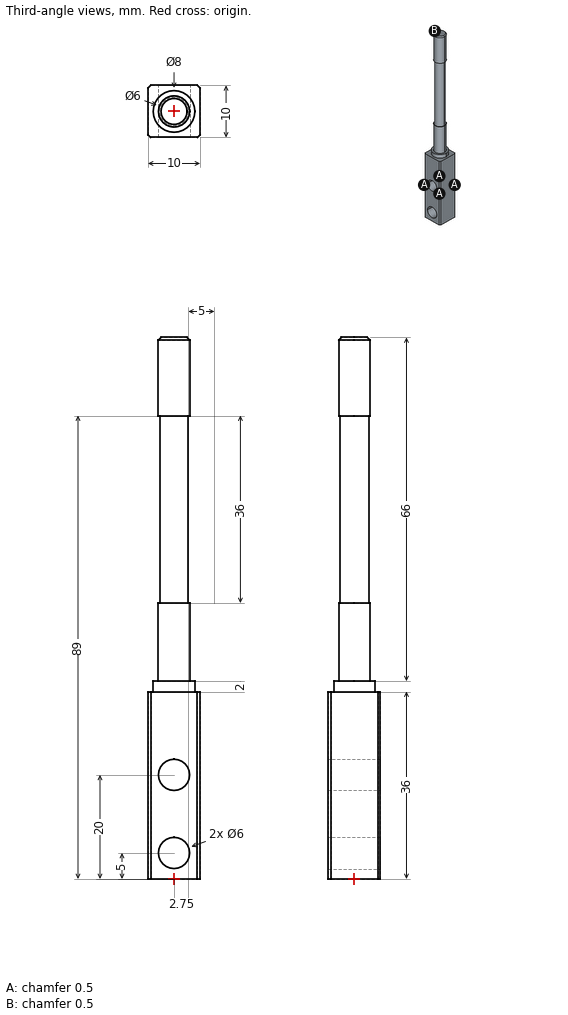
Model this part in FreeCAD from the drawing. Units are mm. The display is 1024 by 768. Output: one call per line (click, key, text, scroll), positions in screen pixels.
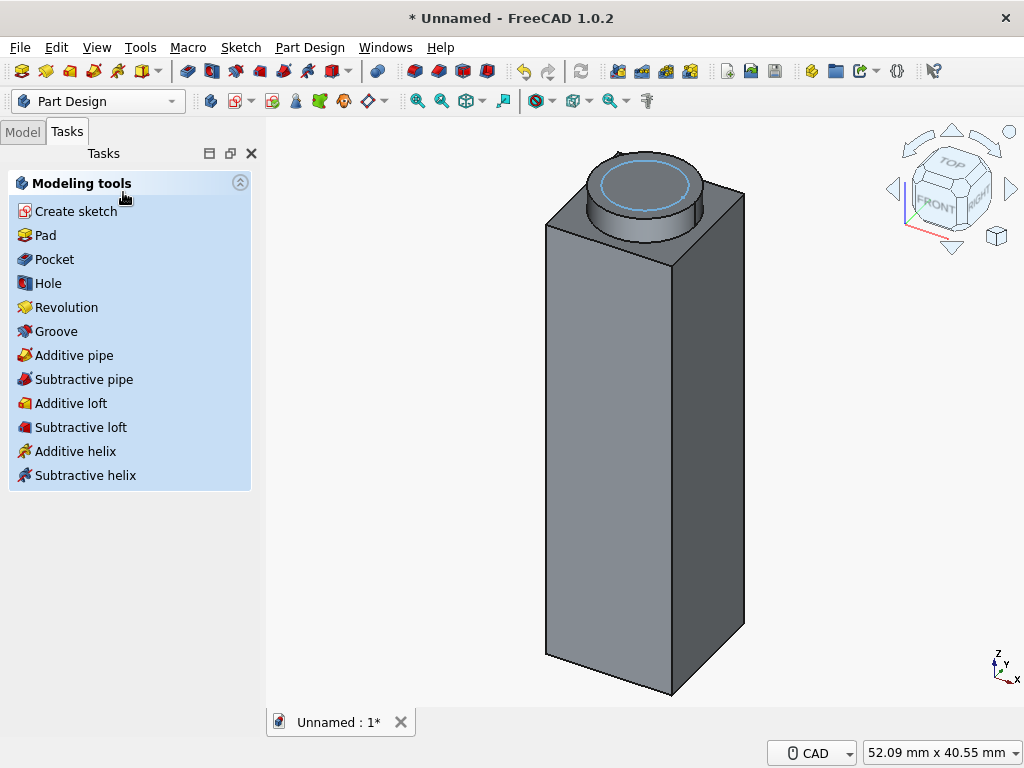
click(22, 72)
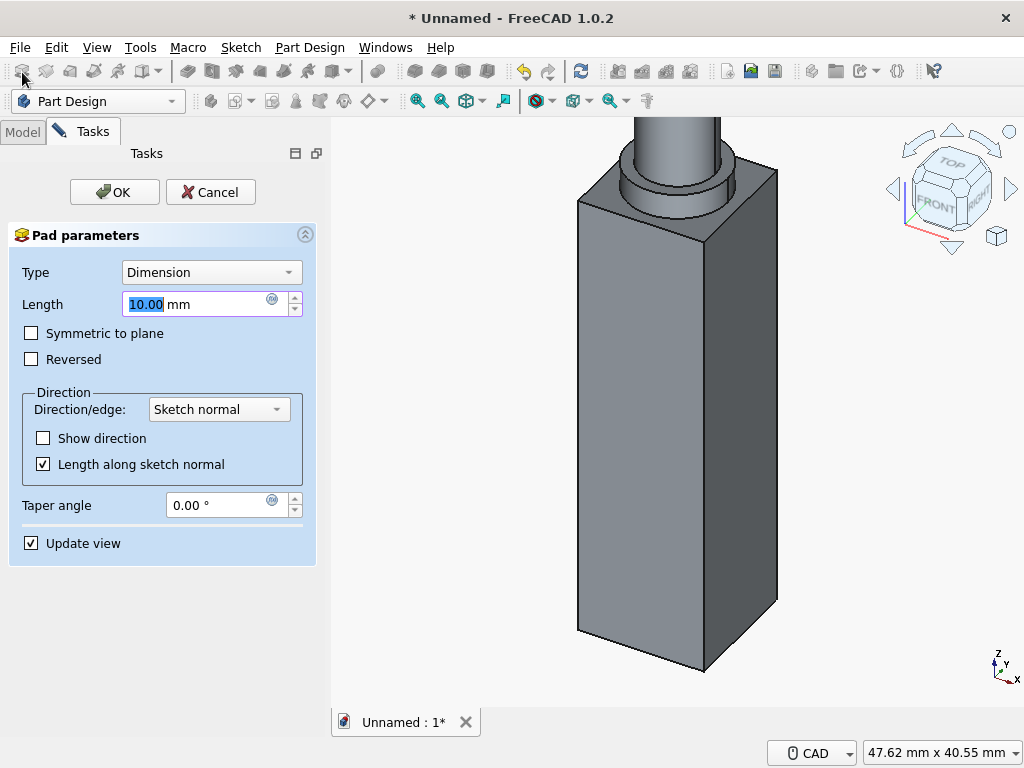
text(66)
key(Tab)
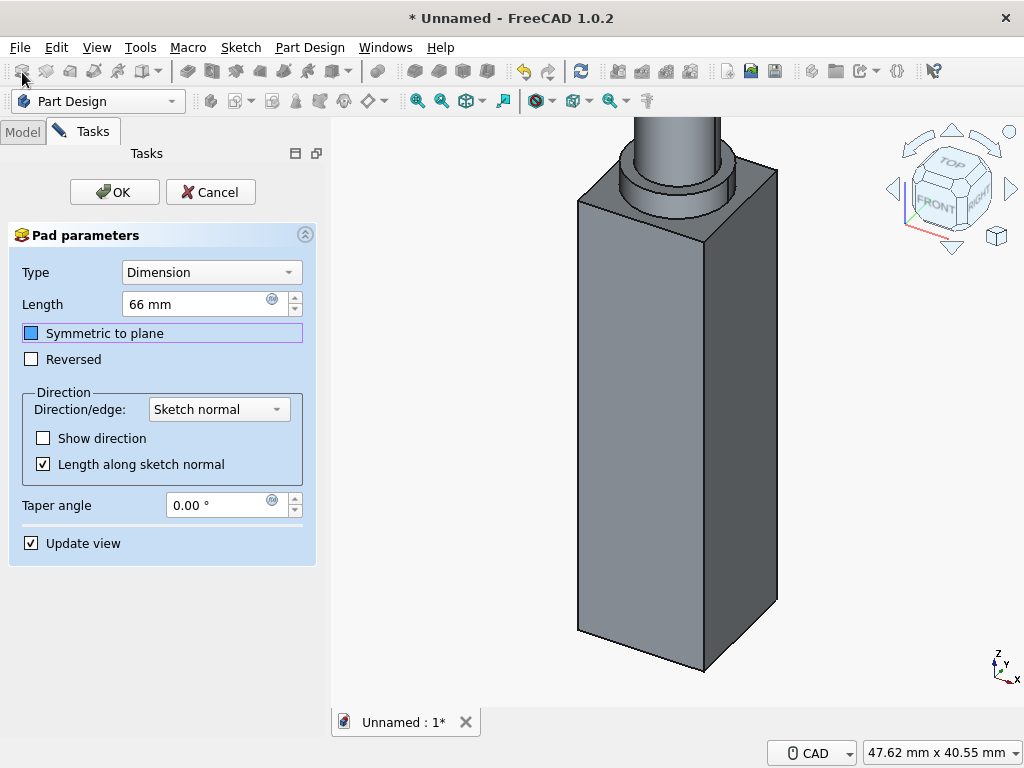
click(115, 192)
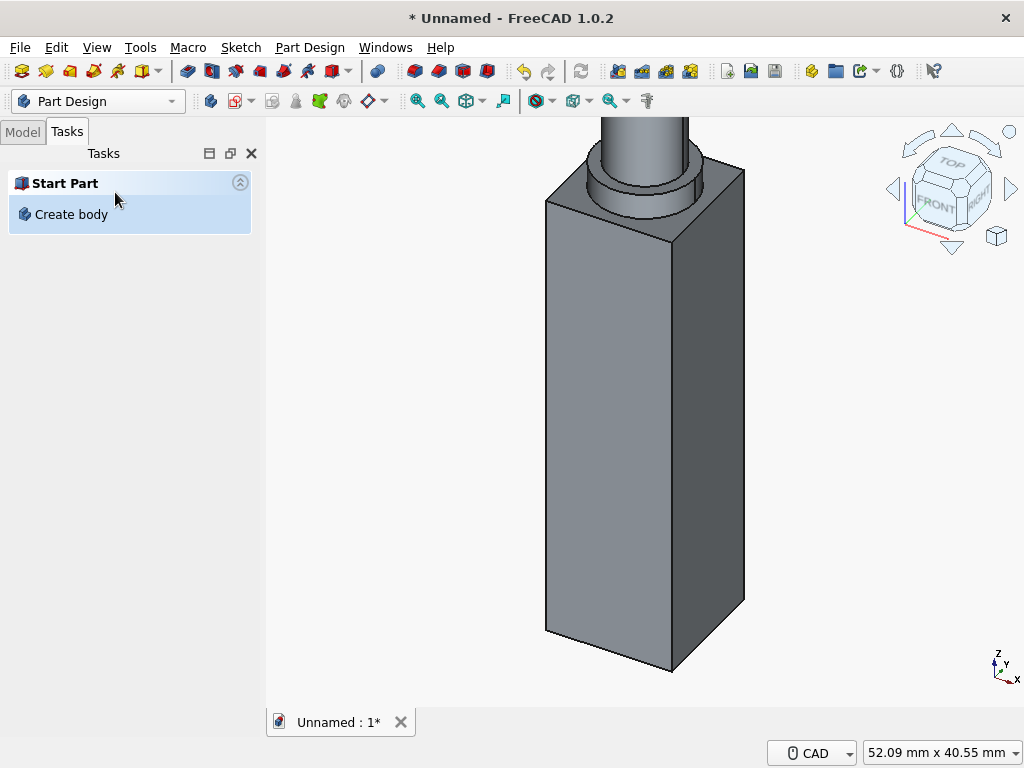
click(418, 102)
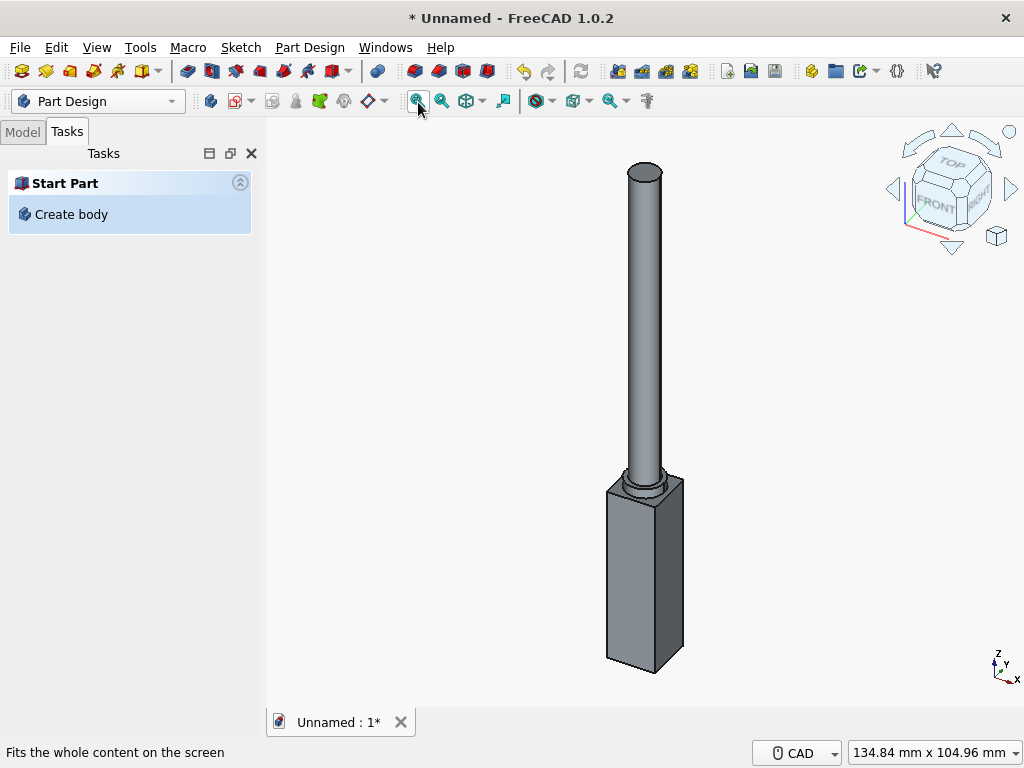
key(4)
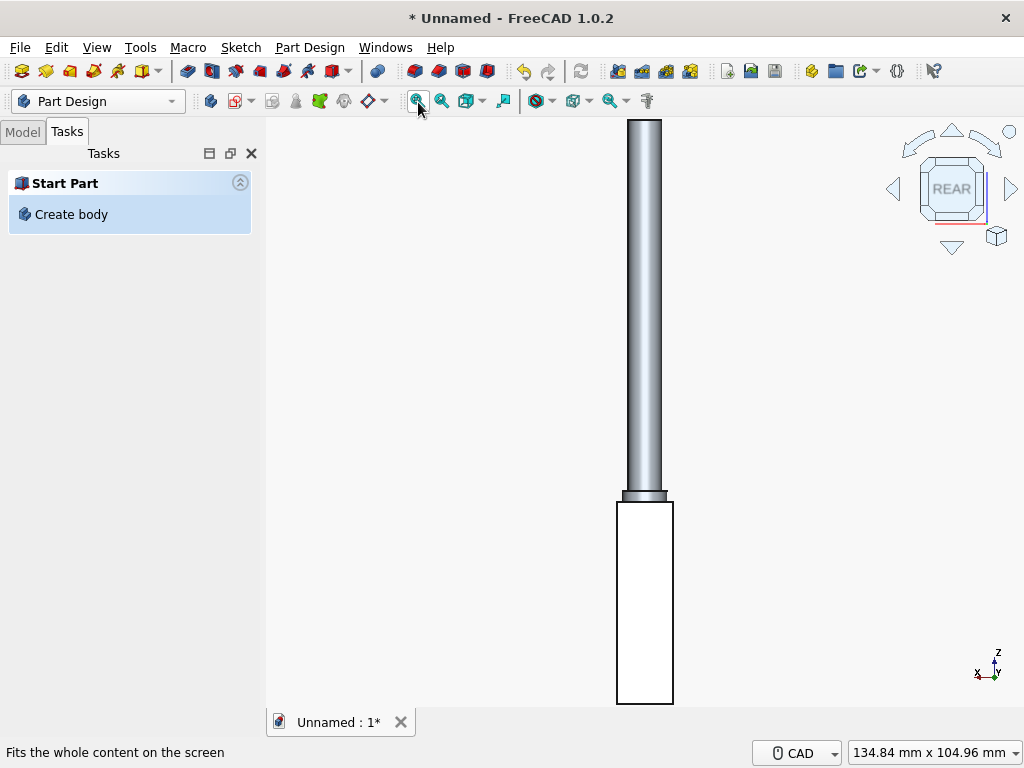
click(645, 544)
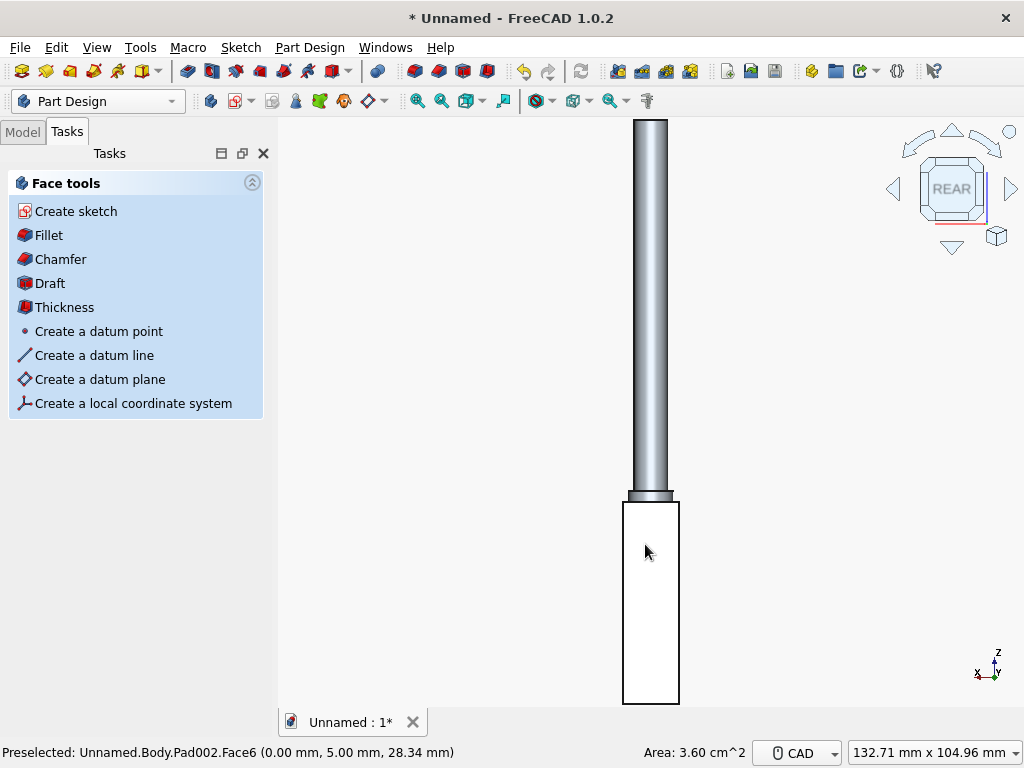
click(236, 102)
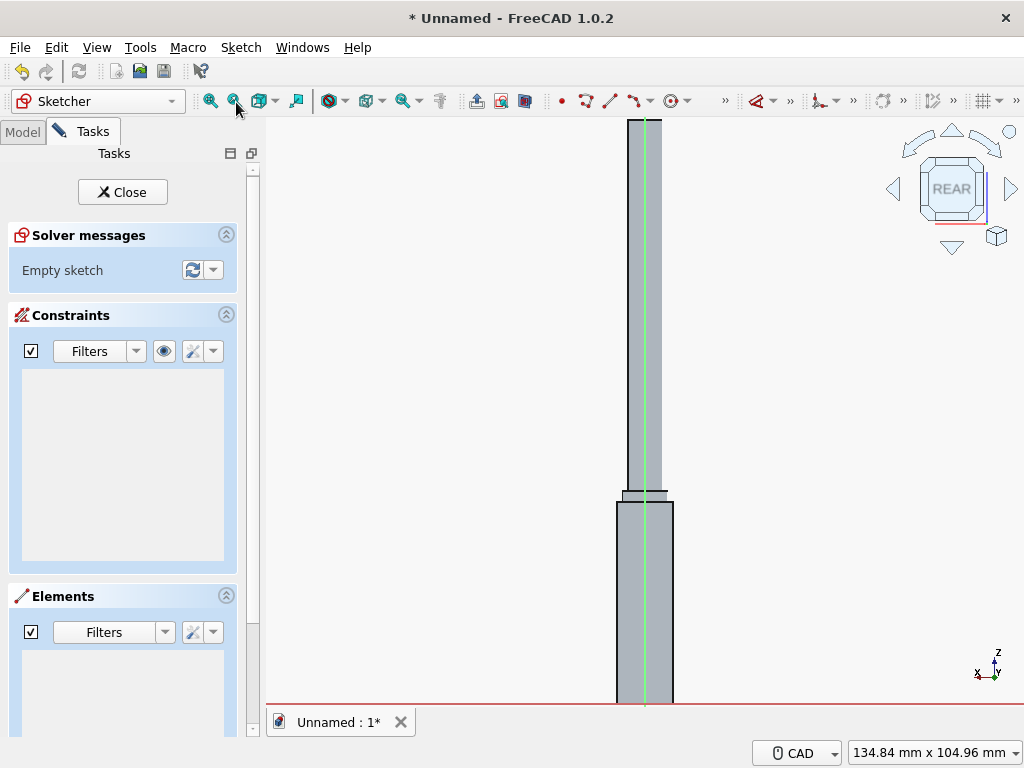
scroll(576, 412, down, 5)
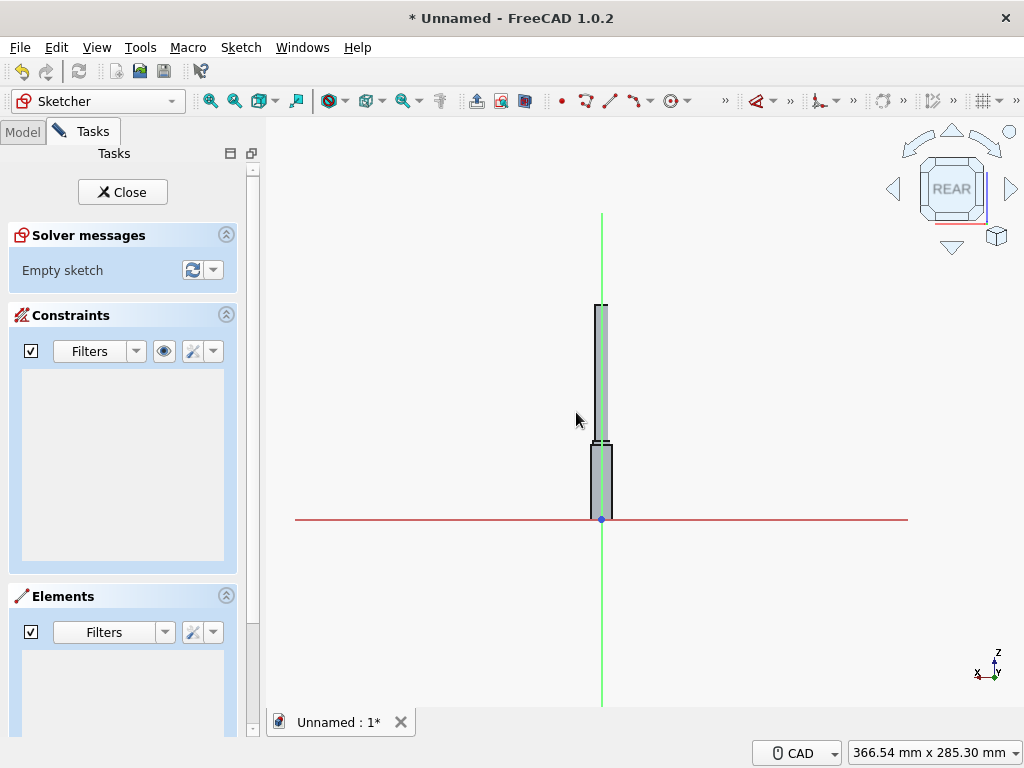
scroll(606, 509, up, 10)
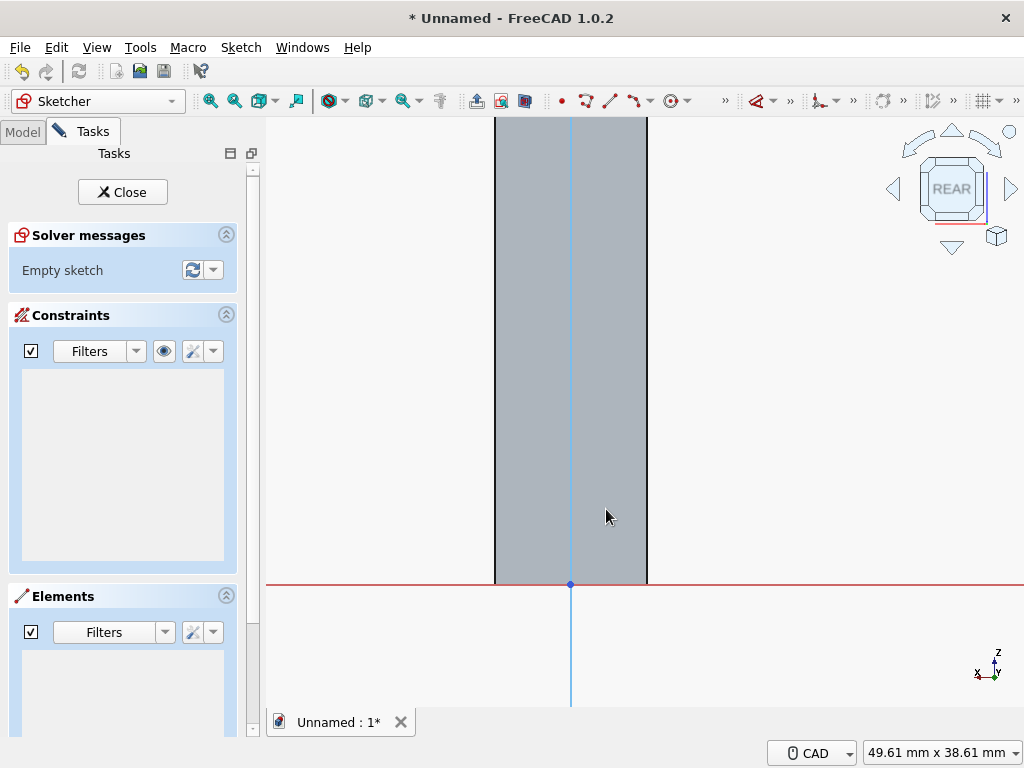
key(g)
key(c)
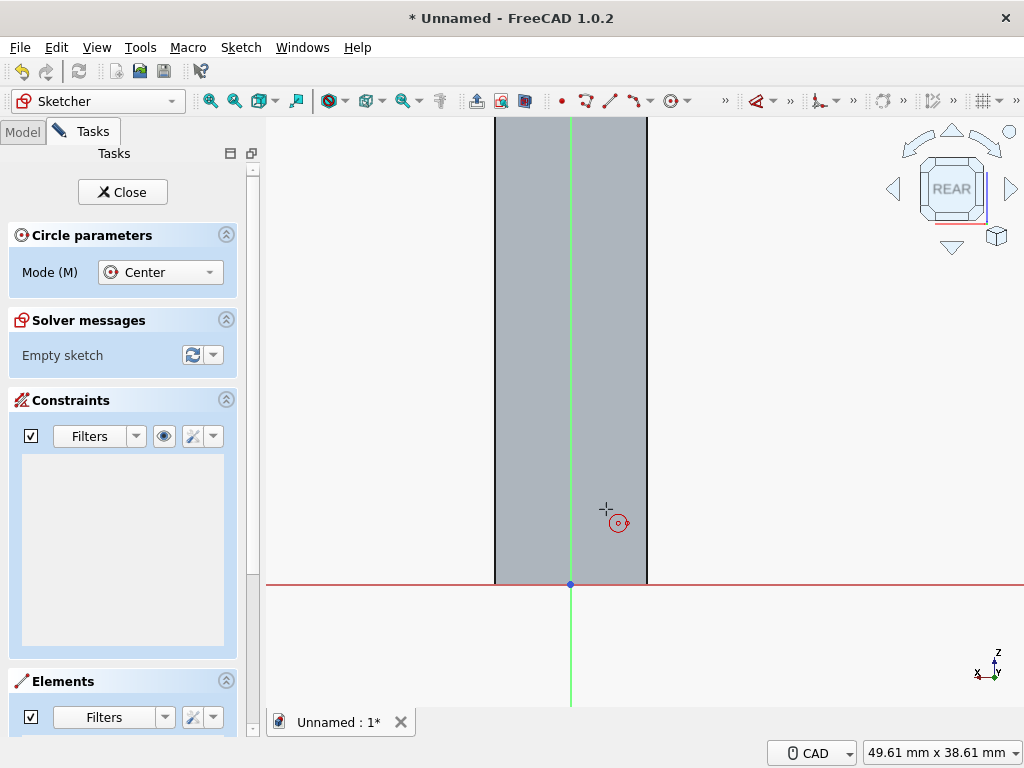
click(571, 509)
click(603, 476)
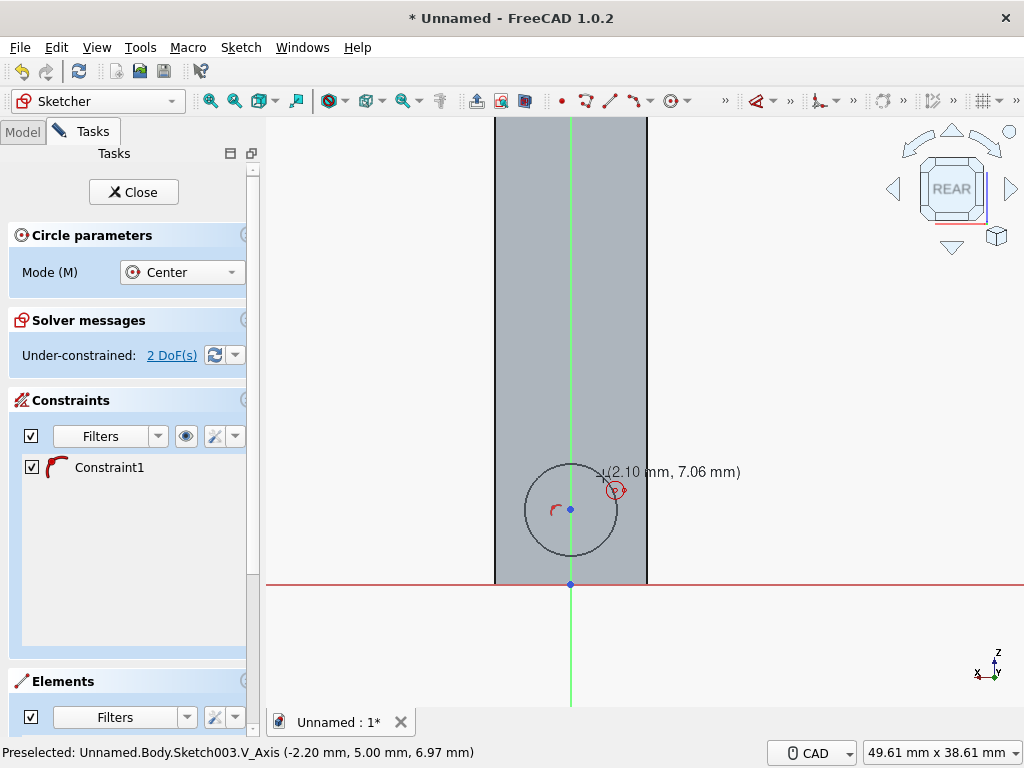
click(571, 279)
click(603, 247)
key(Escape)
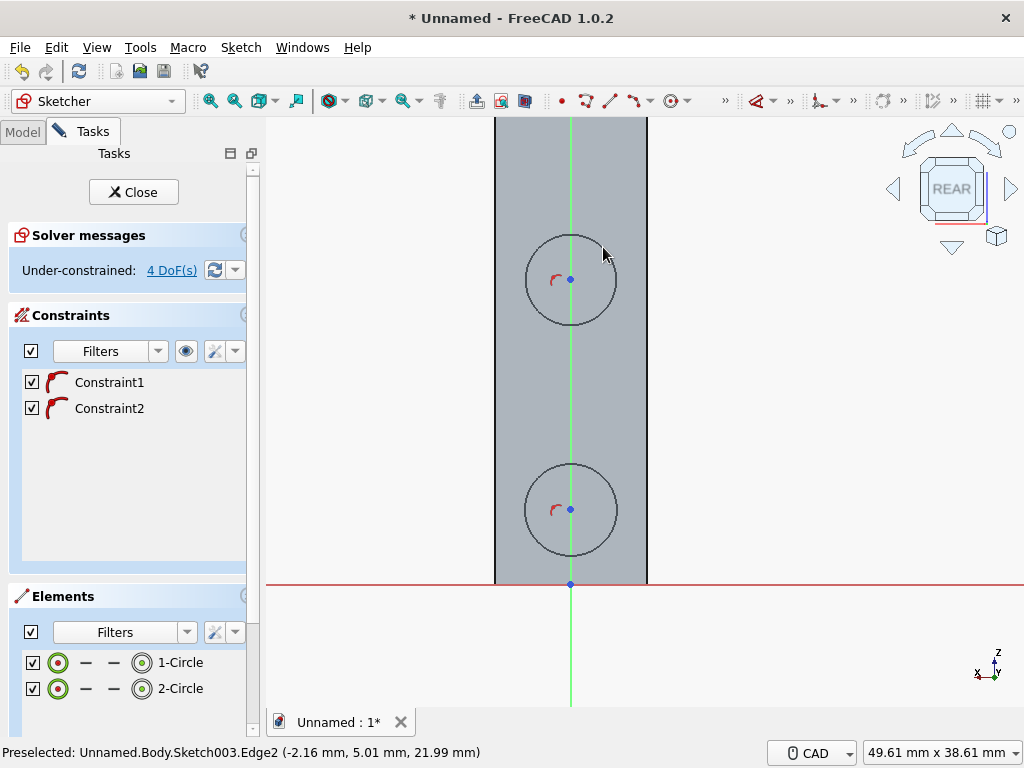
click(603, 477)